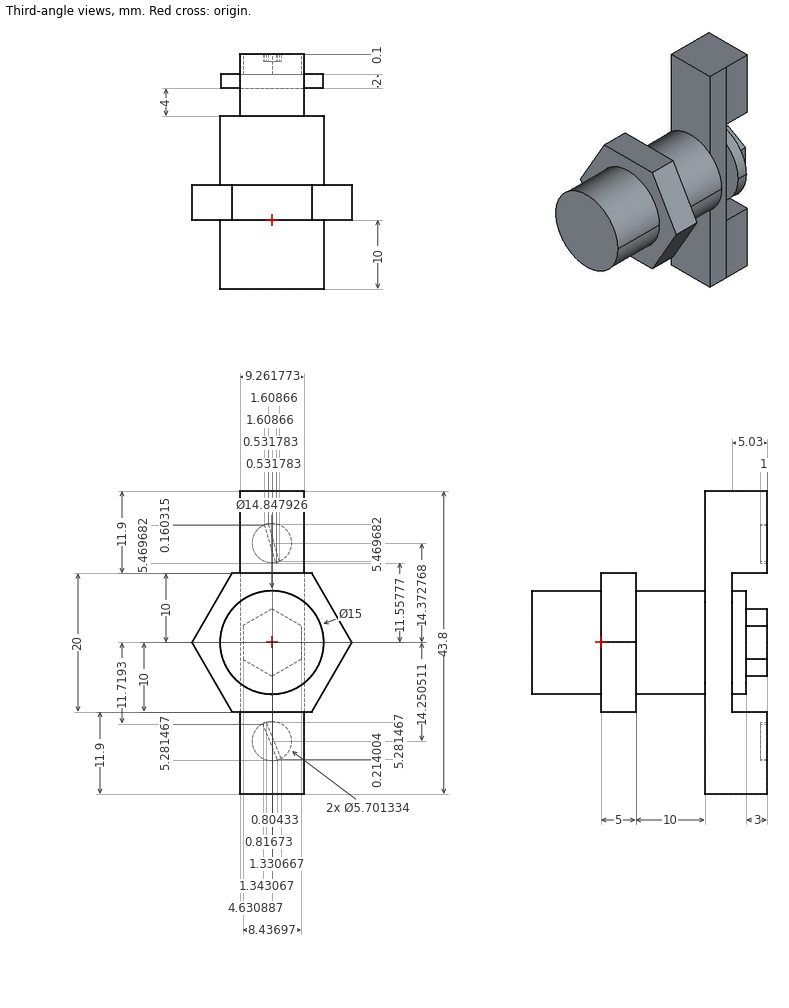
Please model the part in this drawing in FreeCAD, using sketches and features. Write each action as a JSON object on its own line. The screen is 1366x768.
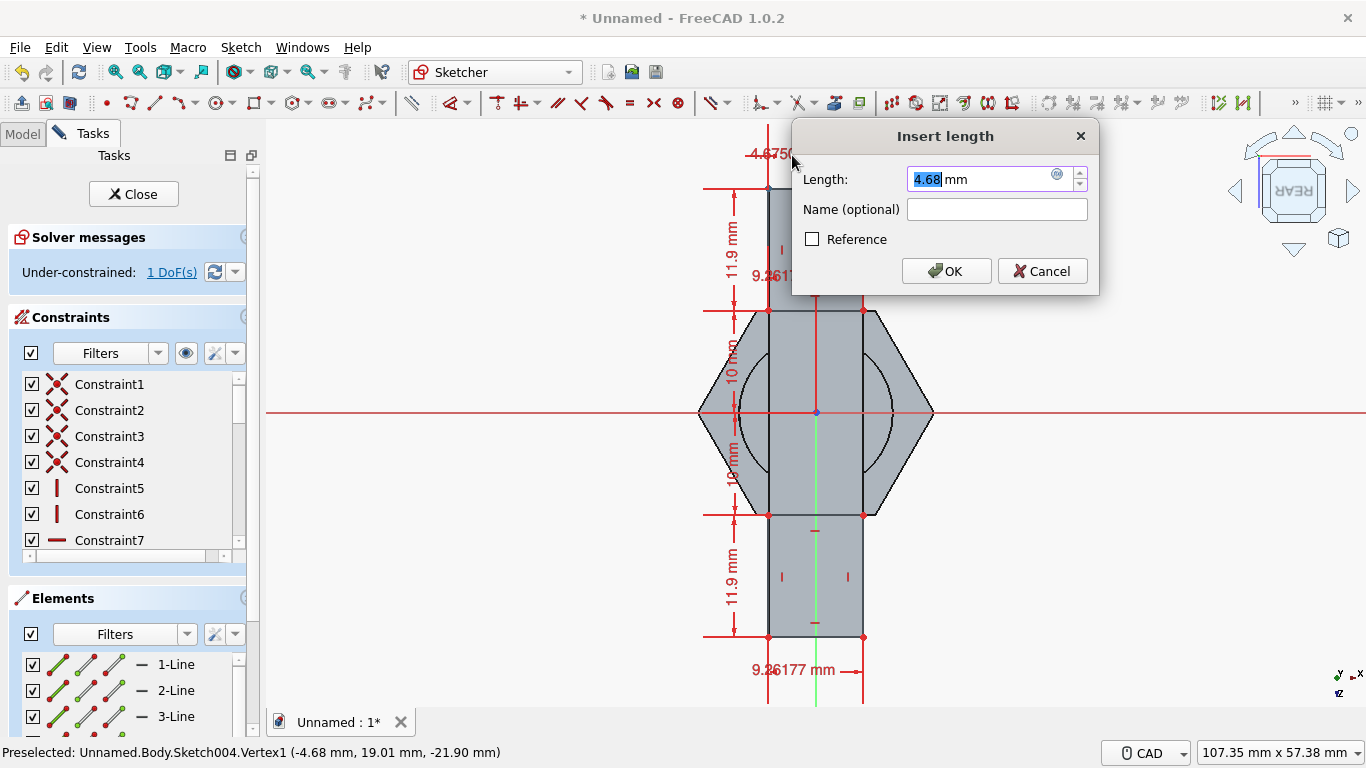
{"action": "type", "text": "4.630887"}
{"action": "key", "text": "Return"}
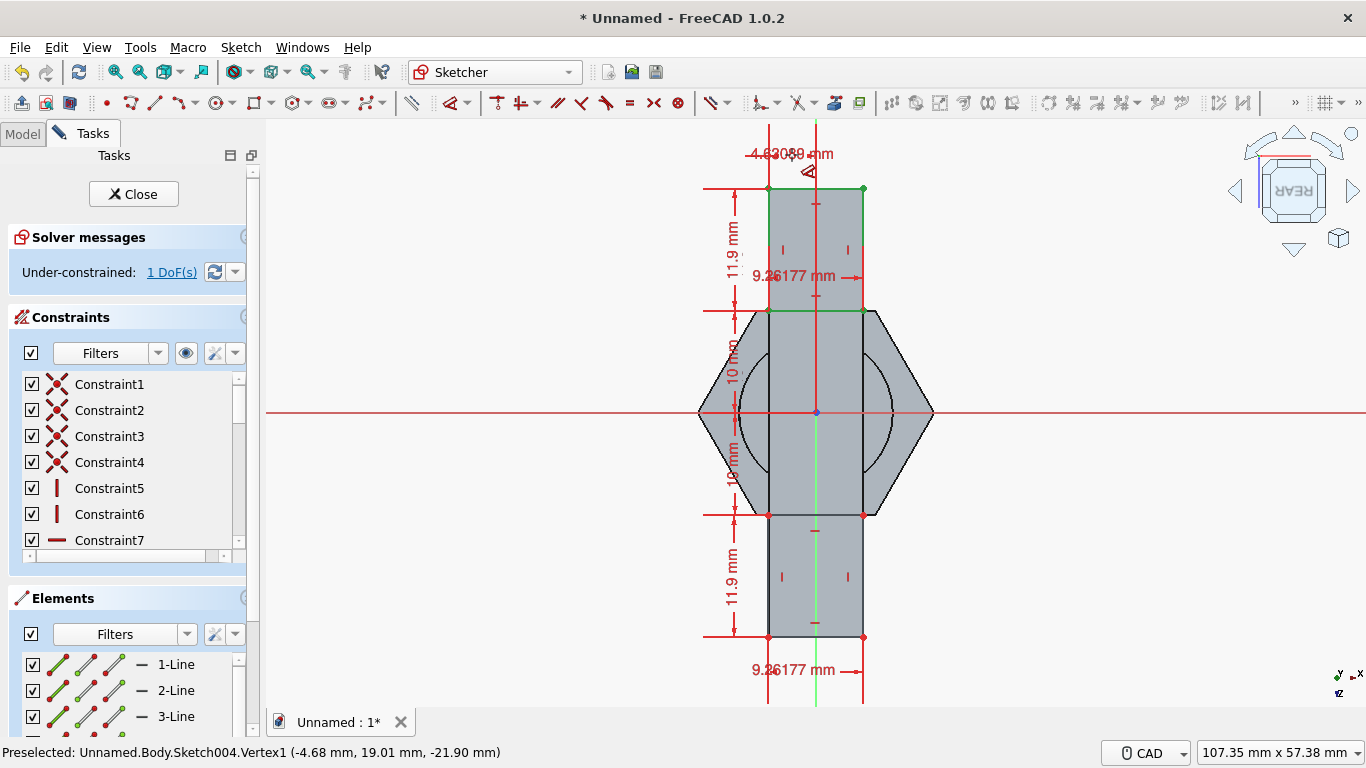
{"action": "left_click", "coordinate": [768, 515]}
{"action": "left_click", "coordinate": [792, 549]}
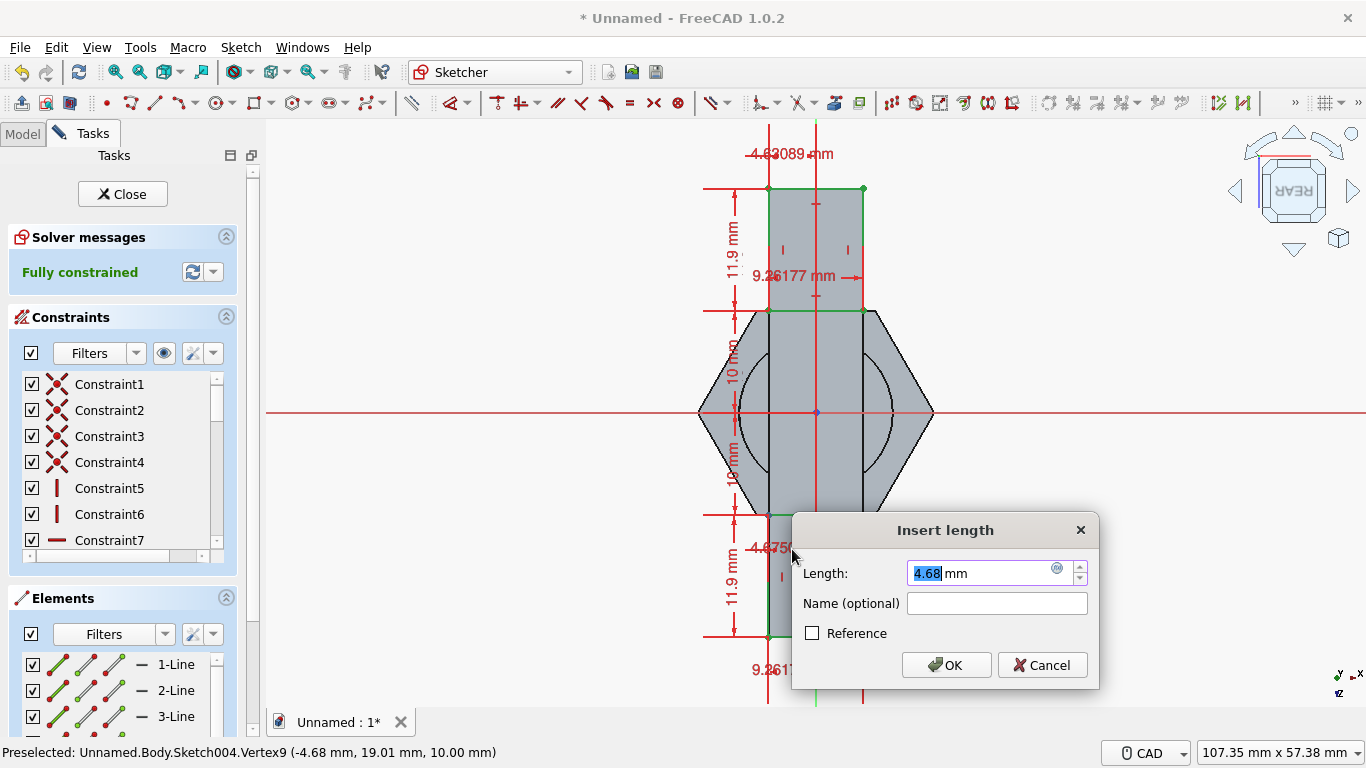
{"action": "type", "text": "4.630887"}
{"action": "key", "text": "Return"}
{"action": "key", "text": "Escape"}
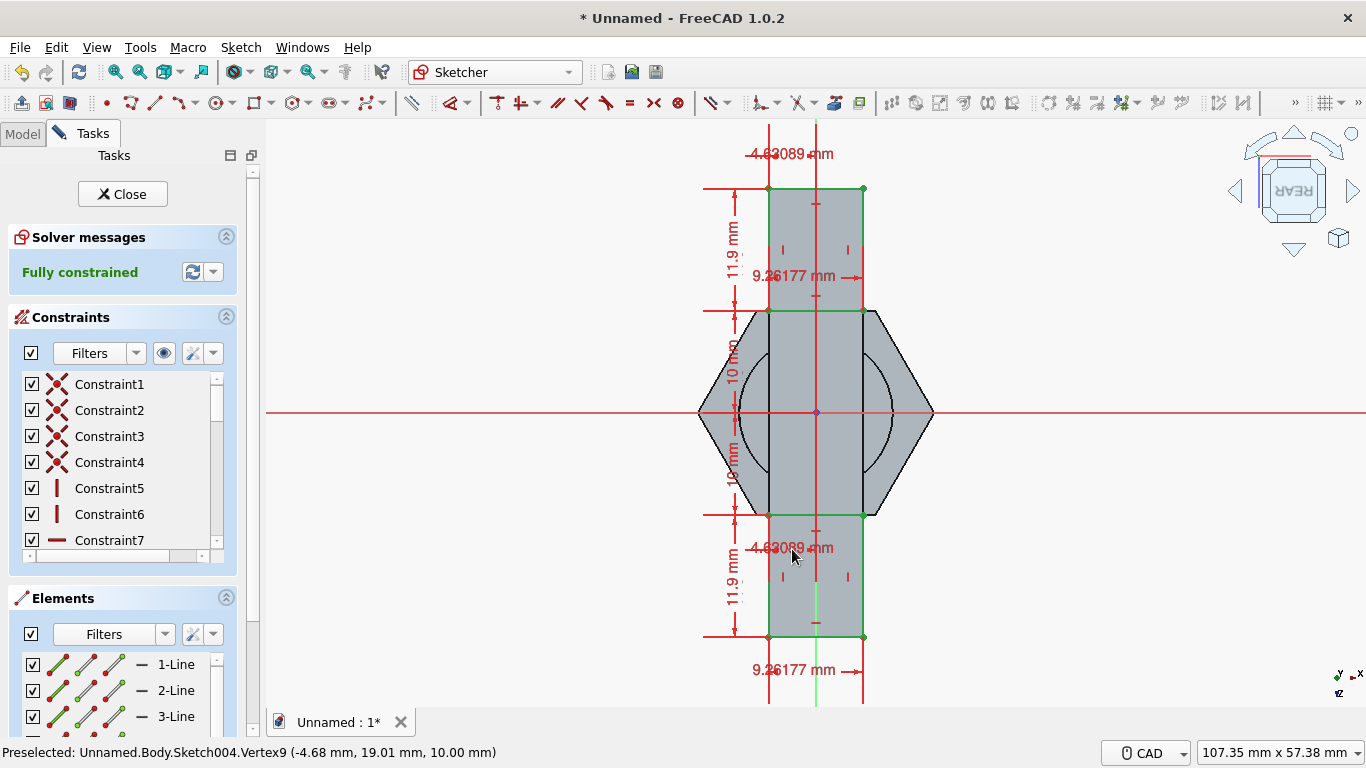
{"action": "left_click", "coordinate": [123, 194]}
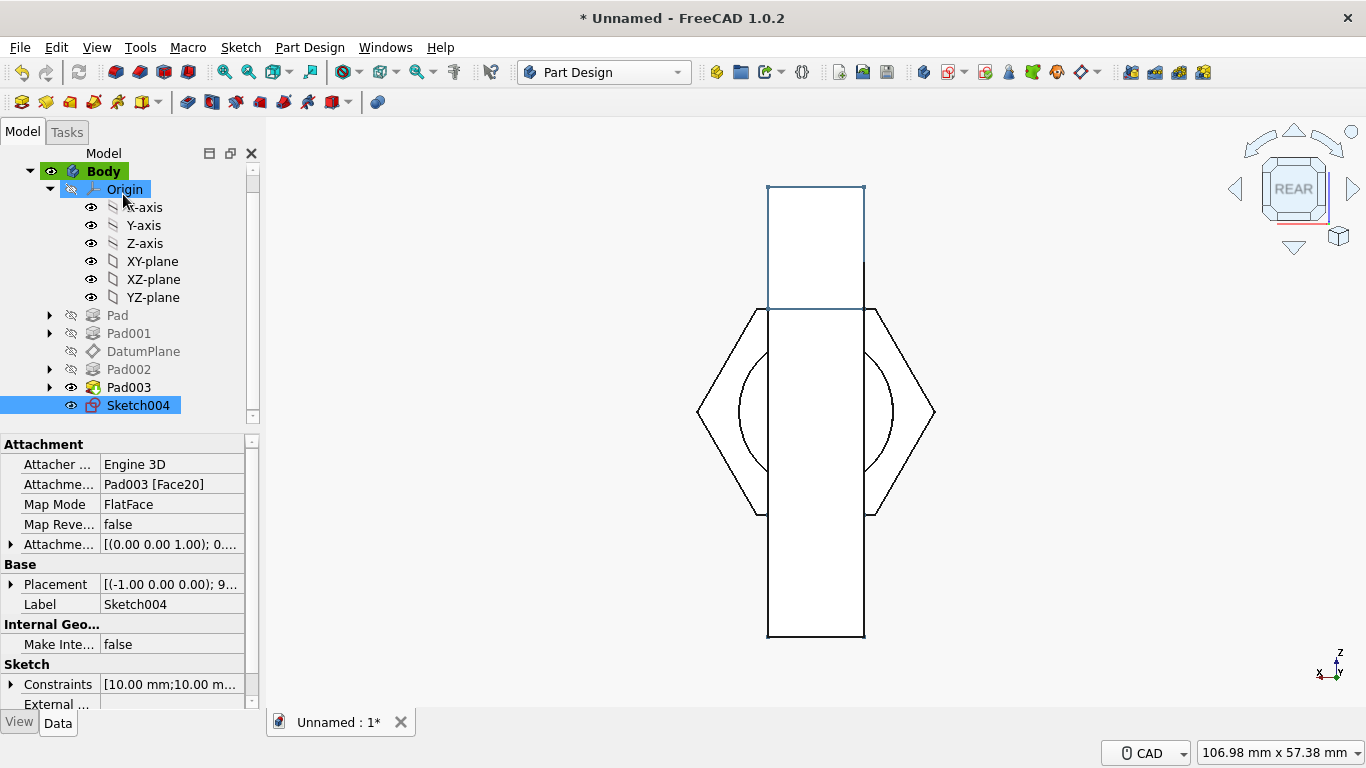
{"action": "left_click", "coordinate": [22, 102]}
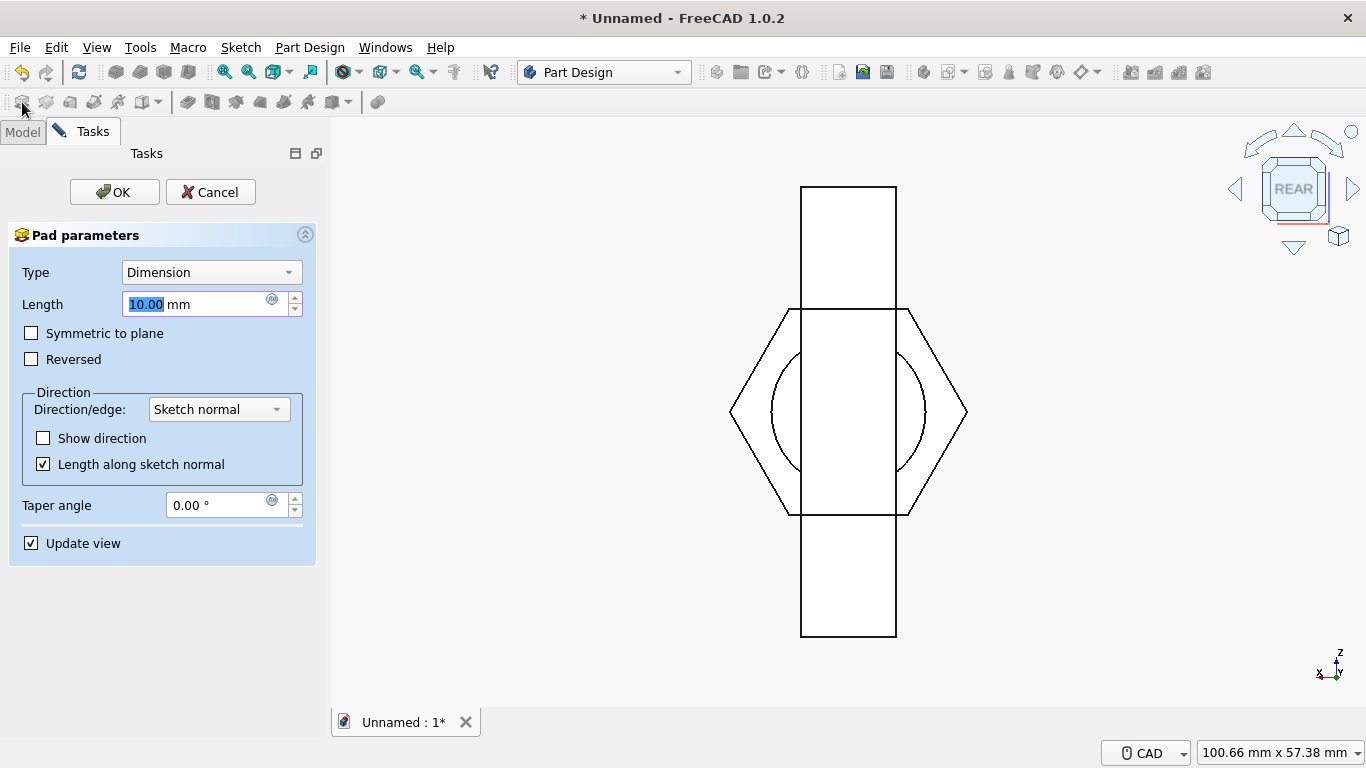
{"action": "type", "text": "5.03"}
{"action": "key", "text": "Tab"}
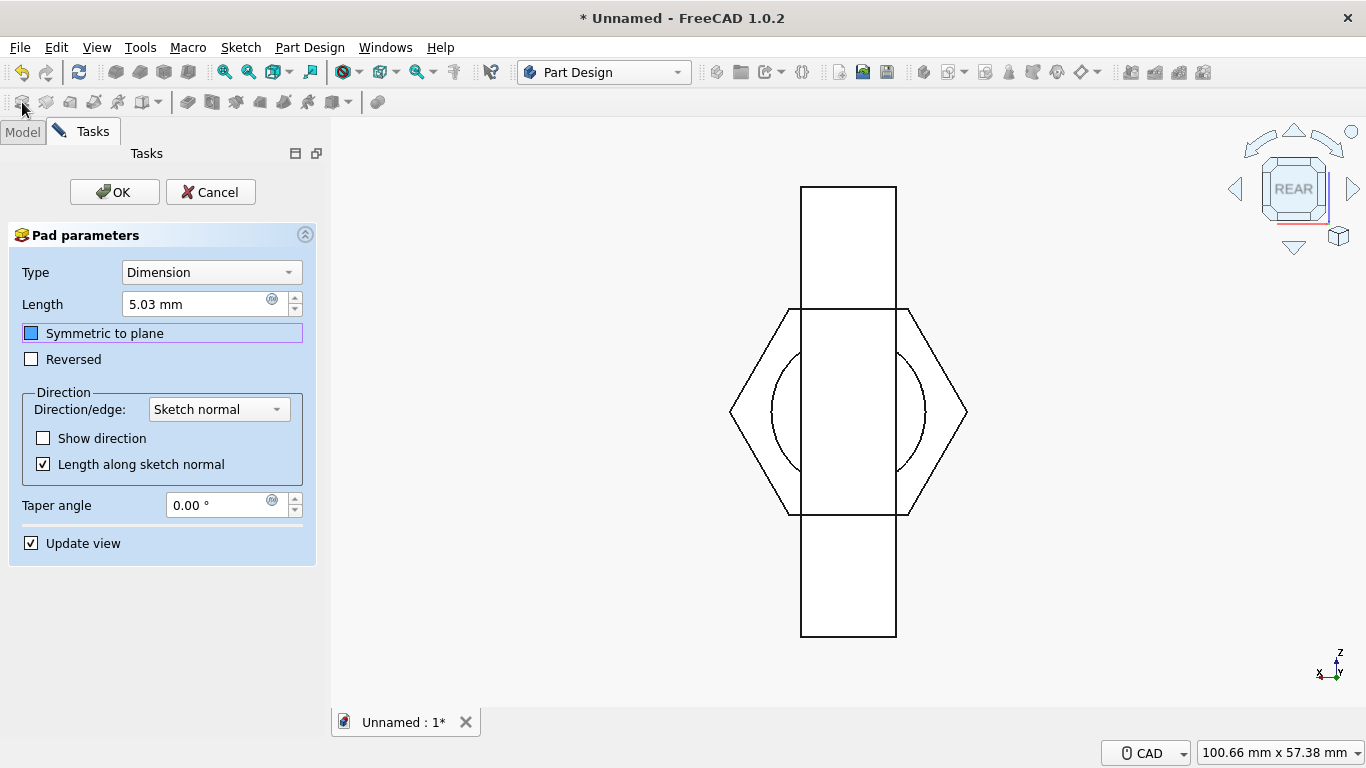
{"action": "left_click", "coordinate": [115, 192]}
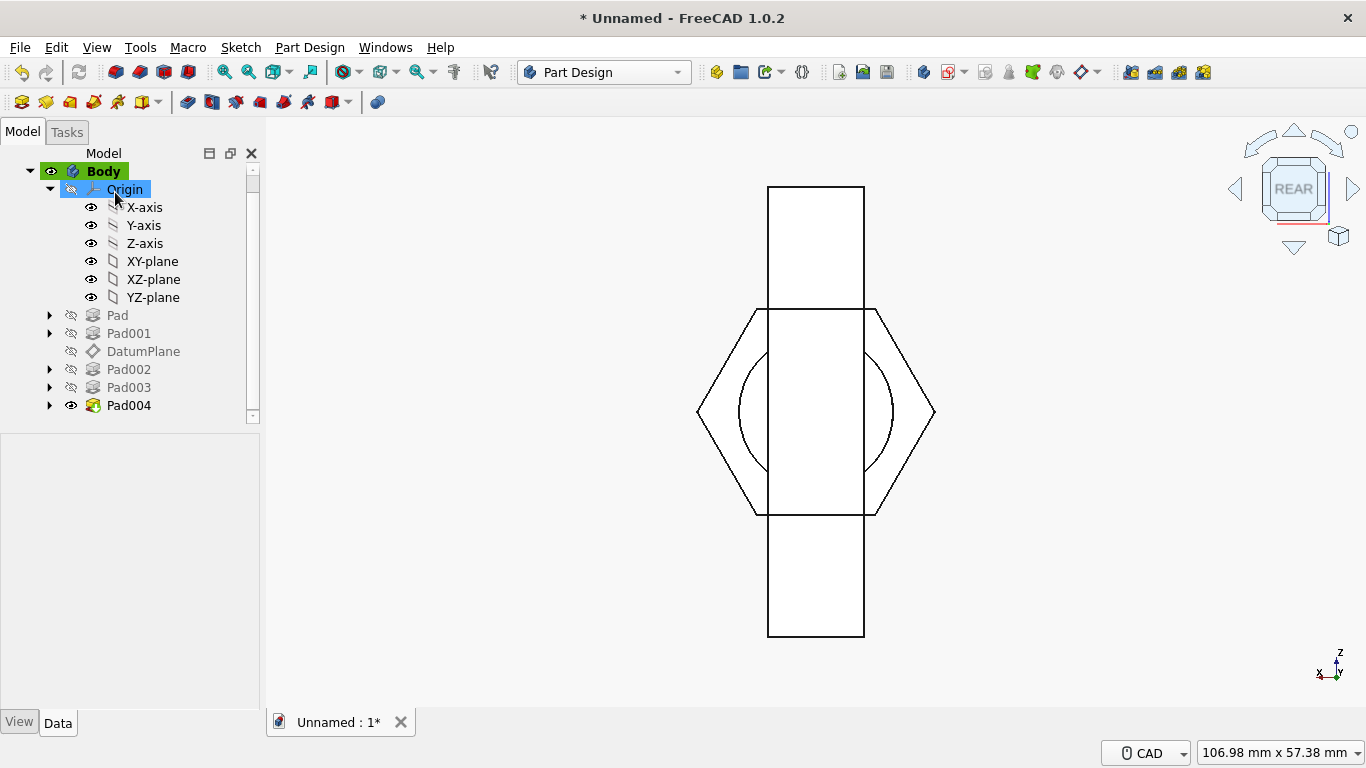
{"action": "left_click", "coordinate": [816, 382]}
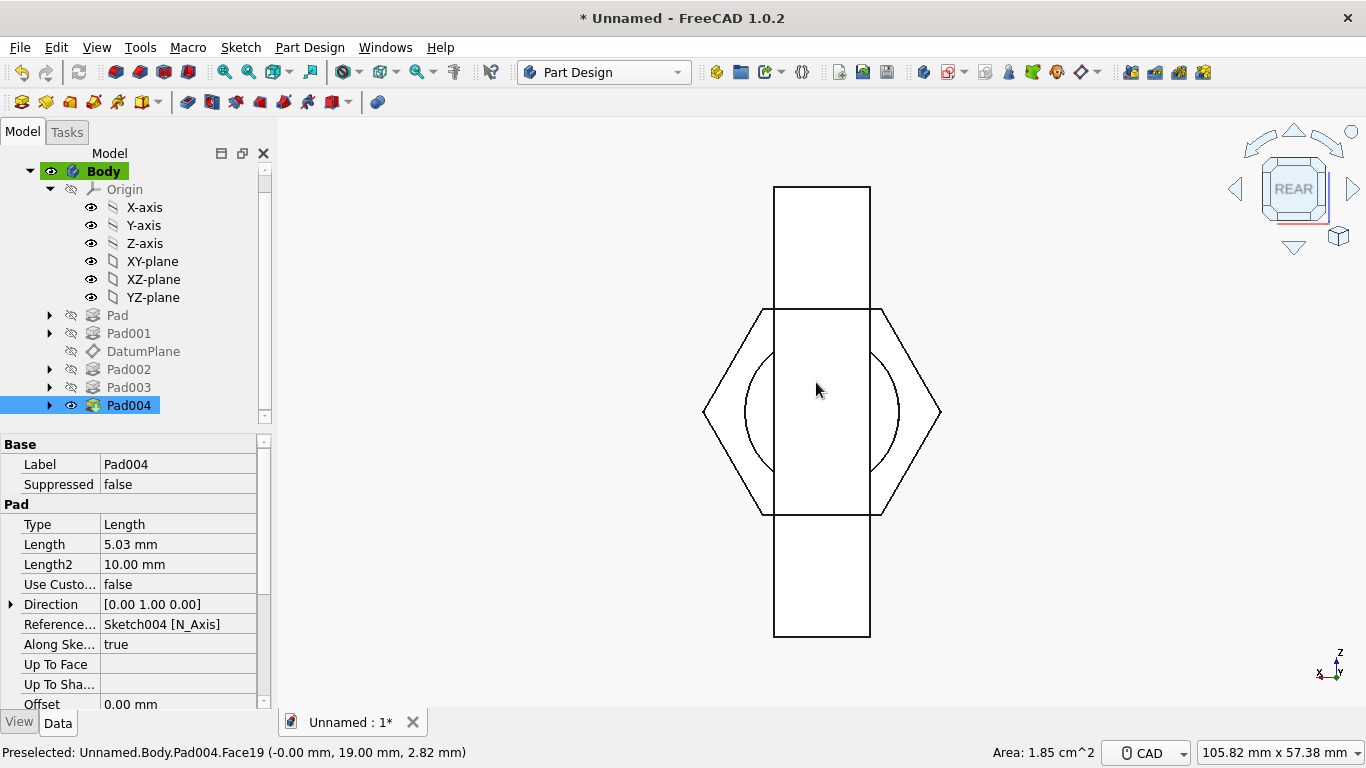
{"action": "left_click", "coordinate": [948, 72]}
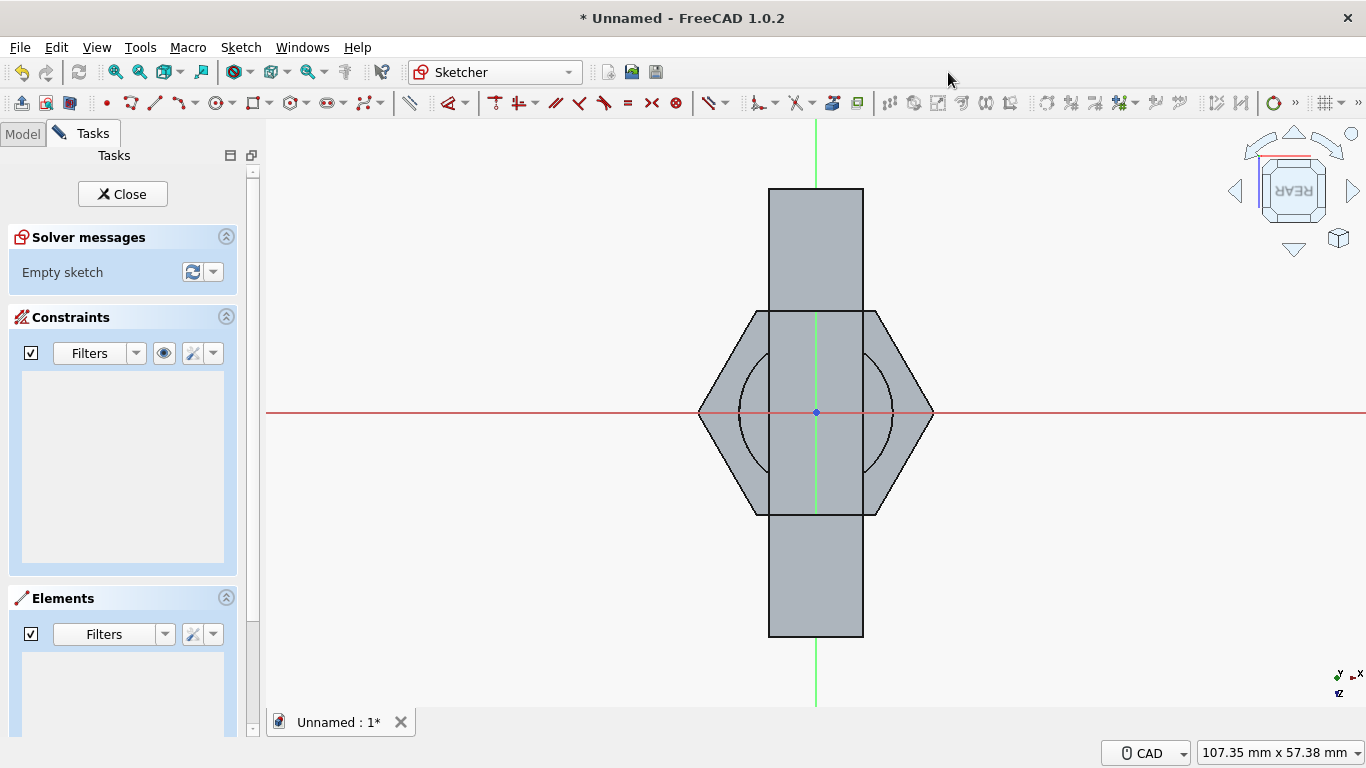
{"action": "scroll", "coordinate": [856, 413], "scroll_direction": "up", "scroll_amount": 5}